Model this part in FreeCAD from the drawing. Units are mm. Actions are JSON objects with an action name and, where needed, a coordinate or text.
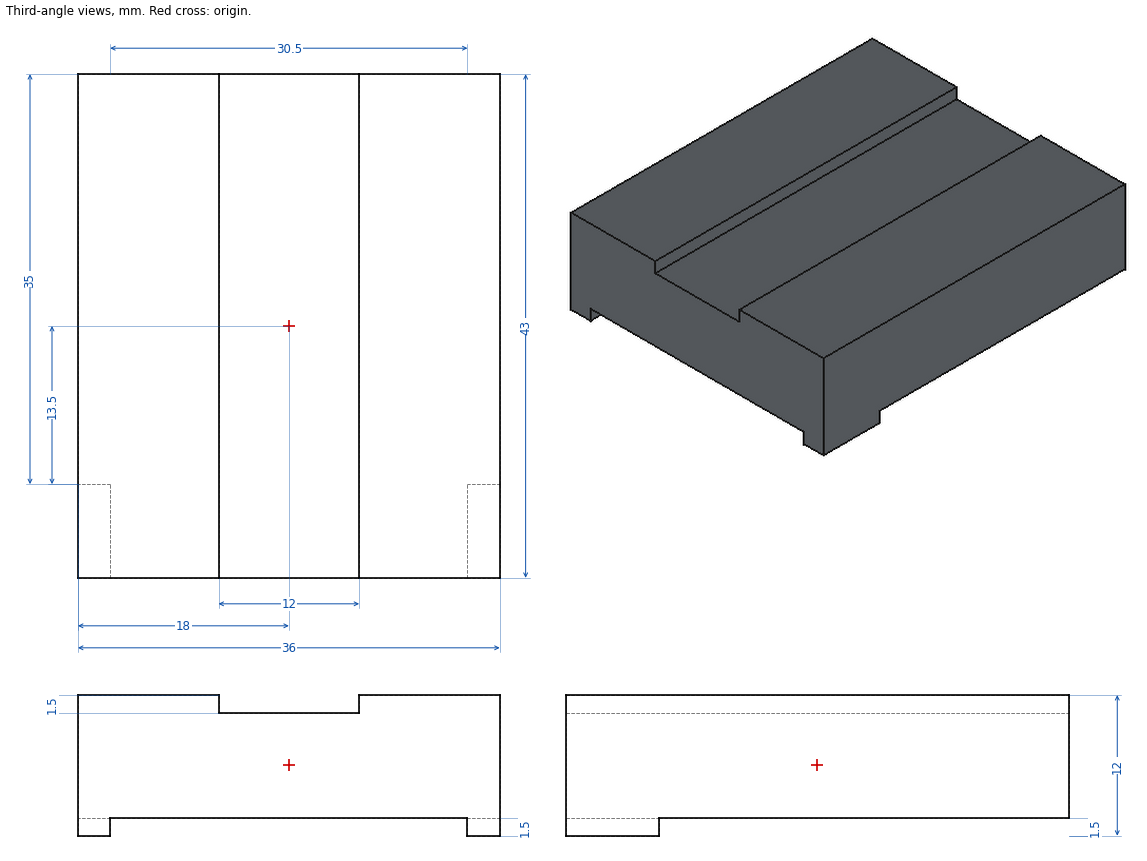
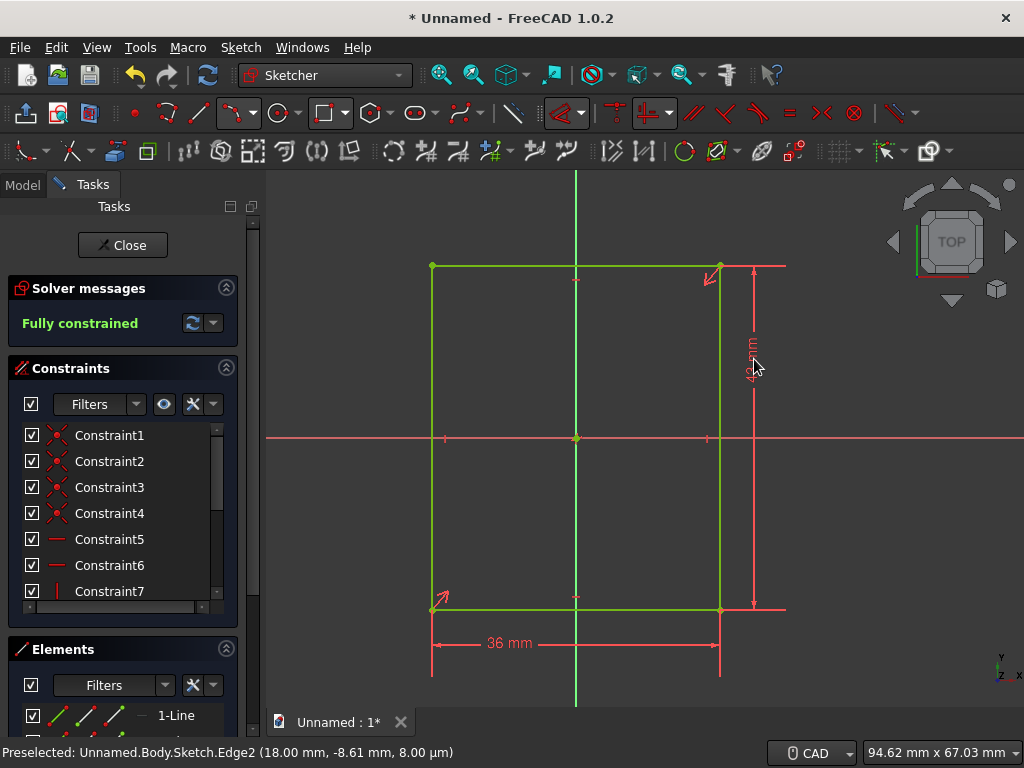
{"action": "left_click", "coordinate": [123, 245]}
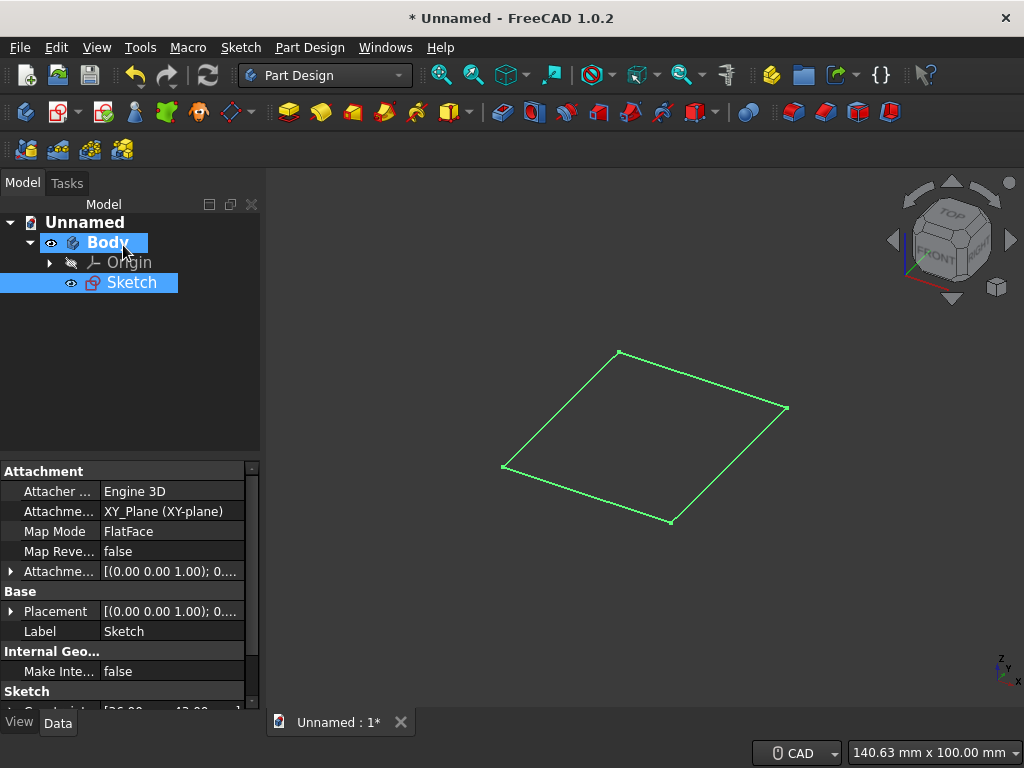
{"action": "left_click", "coordinate": [290, 112]}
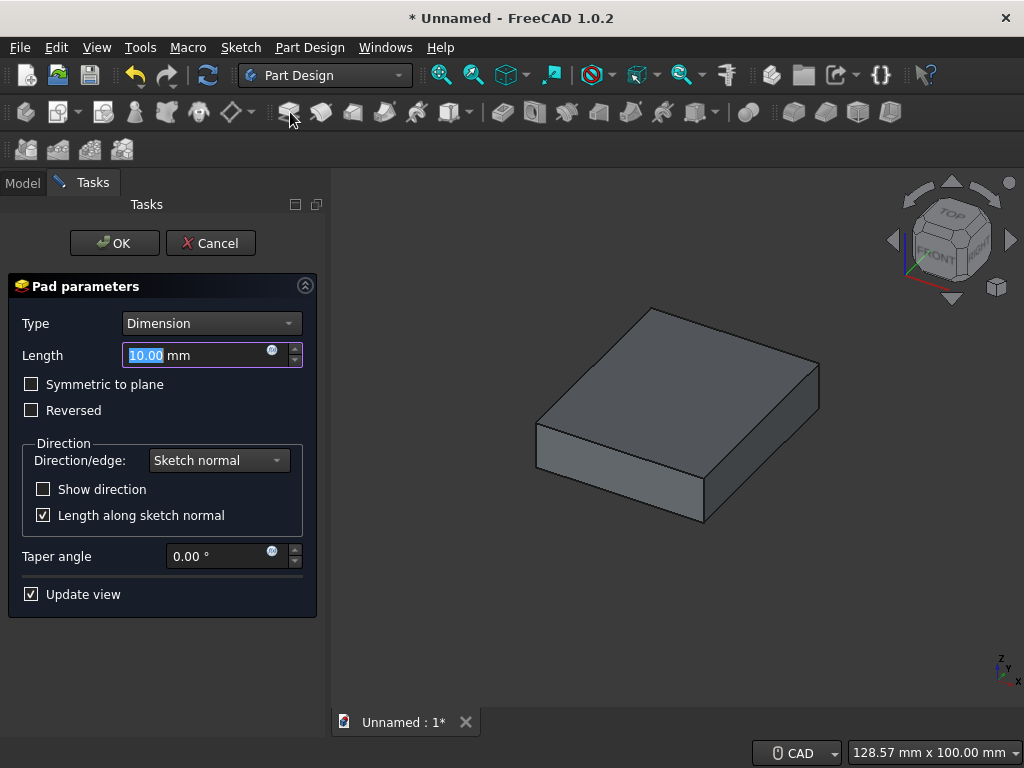
{"action": "type", "text": "12"}
{"action": "key", "text": "Tab"}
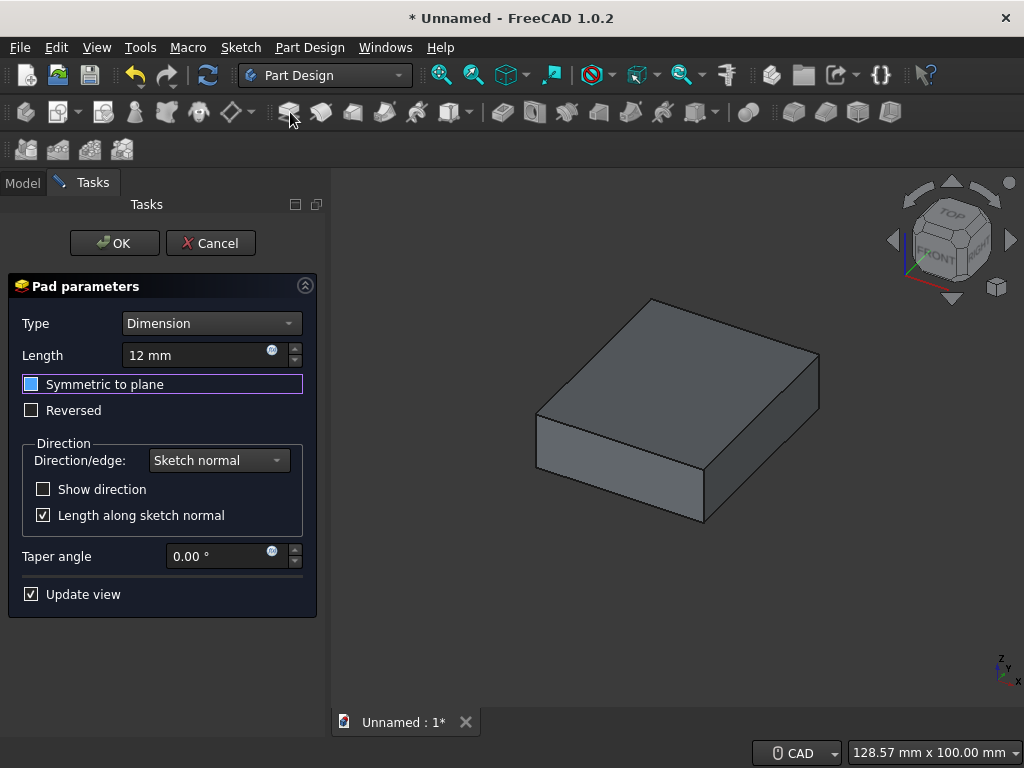
{"action": "left_click", "coordinate": [30, 384]}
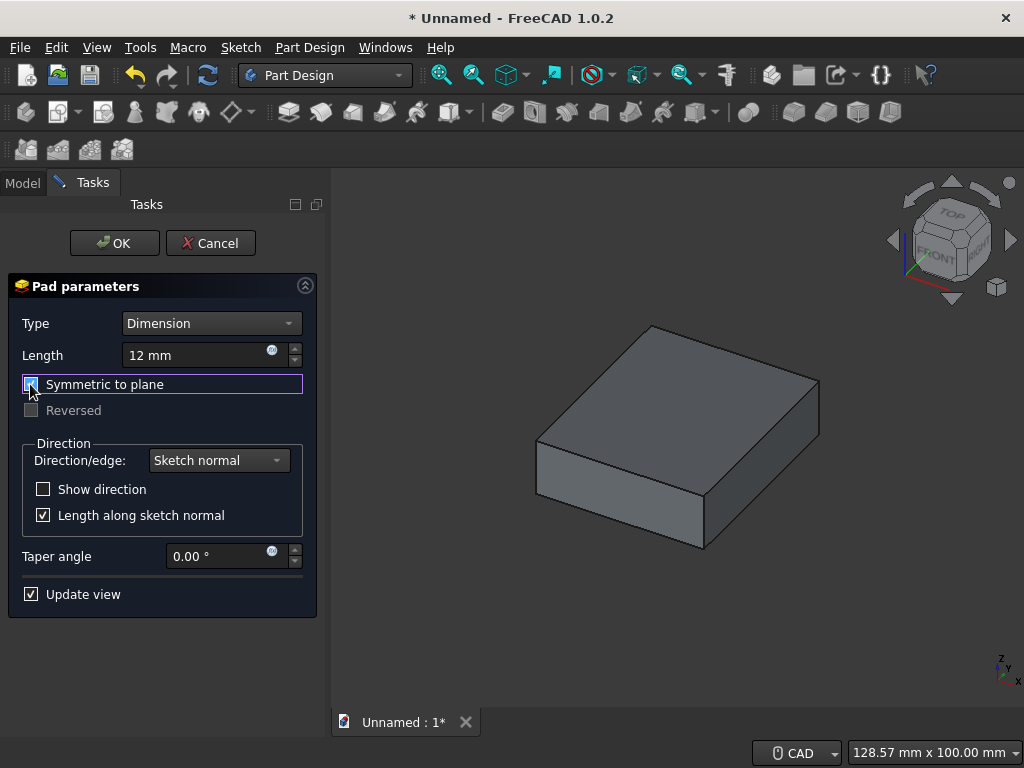
{"action": "left_click", "coordinate": [115, 243]}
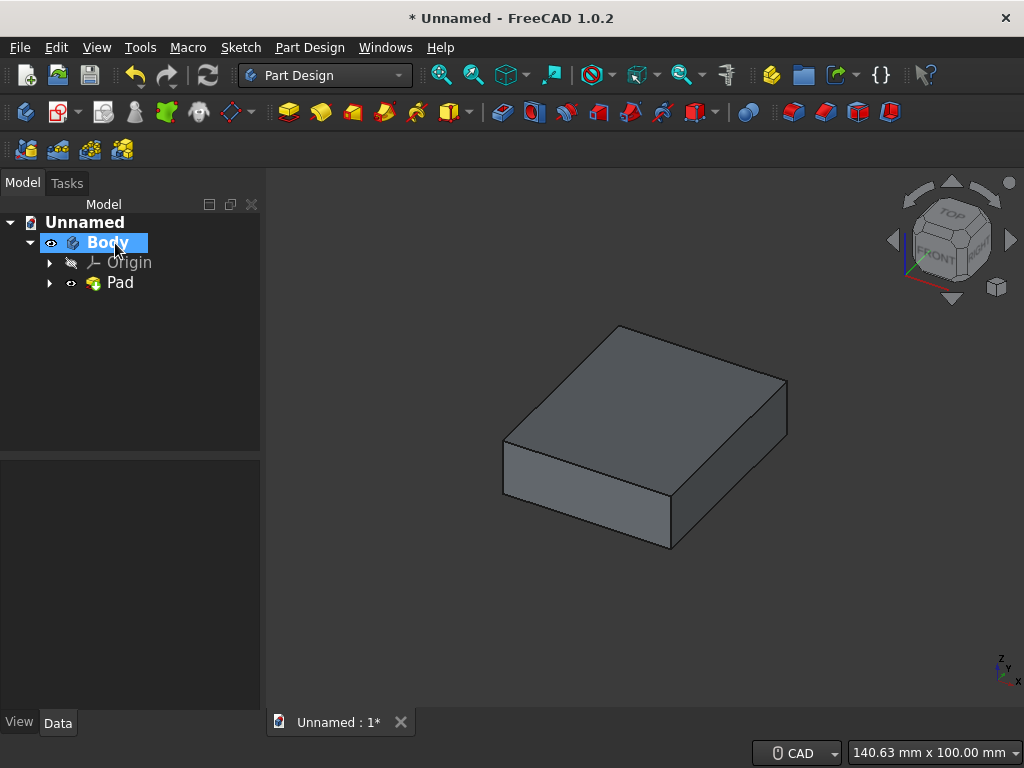
{"action": "key", "text": "v f"}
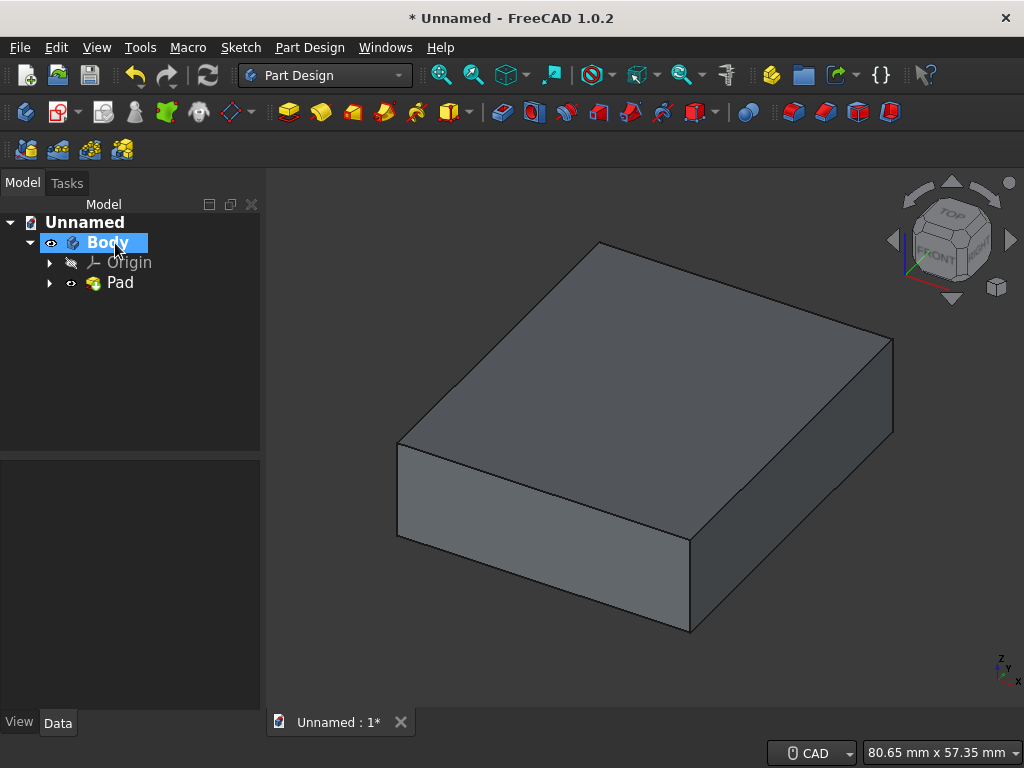
{"action": "left_click", "coordinate": [645, 390]}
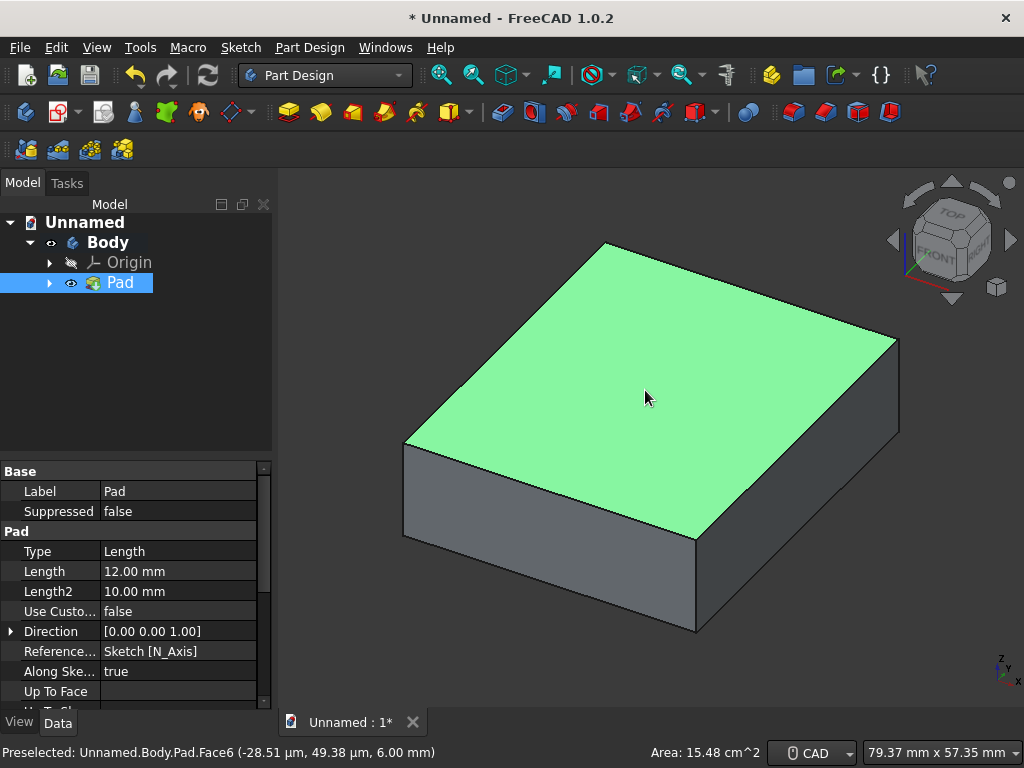
{"action": "left_click", "coordinate": [58, 112]}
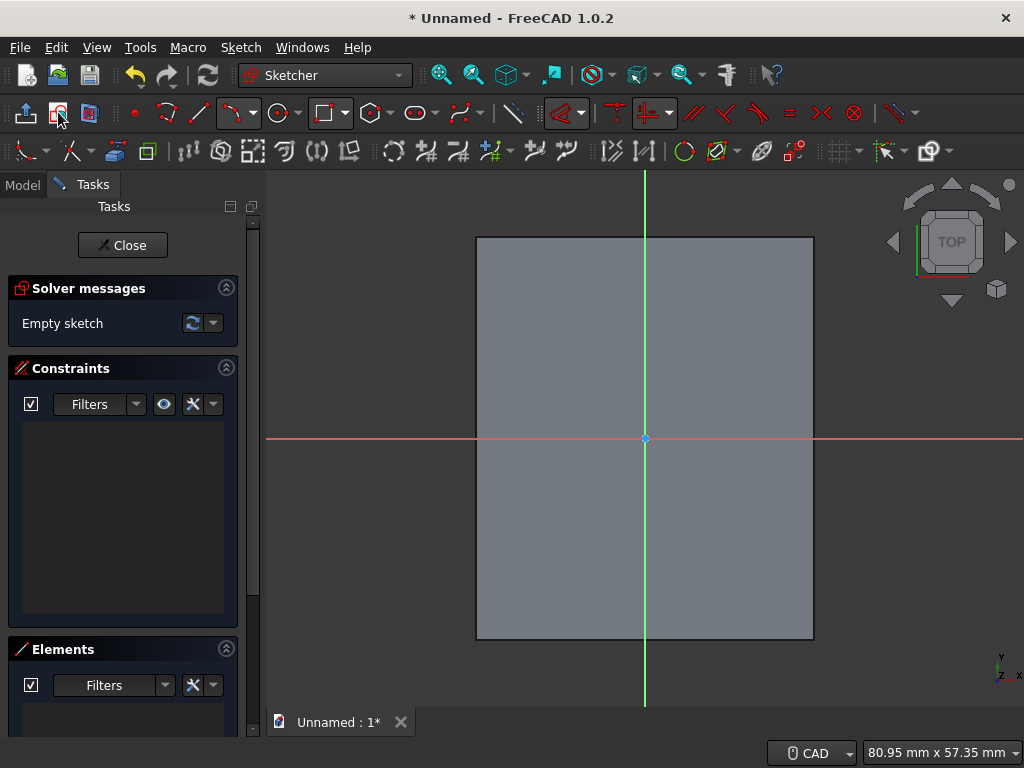
{"action": "key", "text": "g v"}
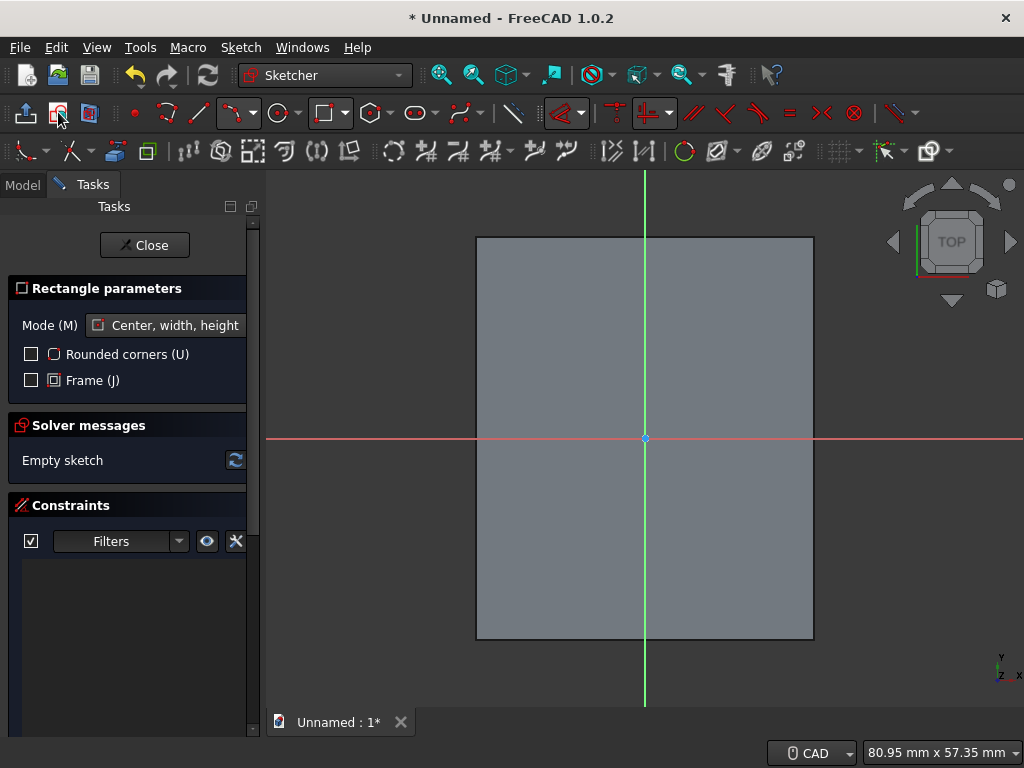
{"action": "left_click", "coordinate": [645, 438]}
{"action": "left_click", "coordinate": [701, 237]}
{"action": "key", "text": "Escape"}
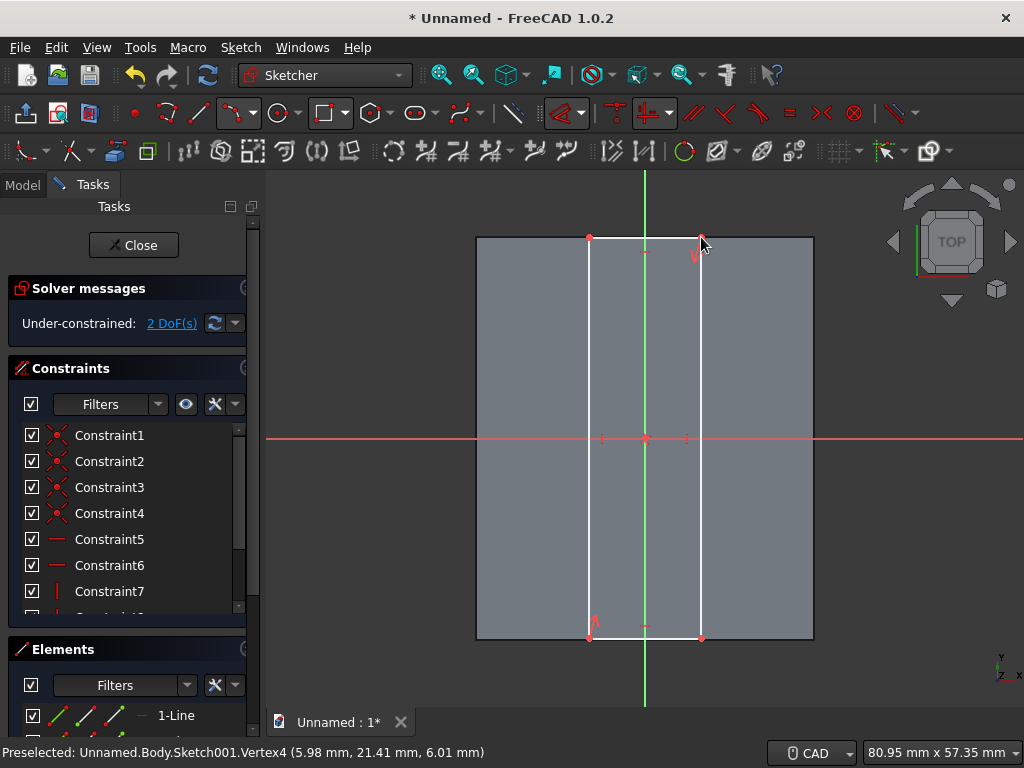
{"action": "key", "text": "d"}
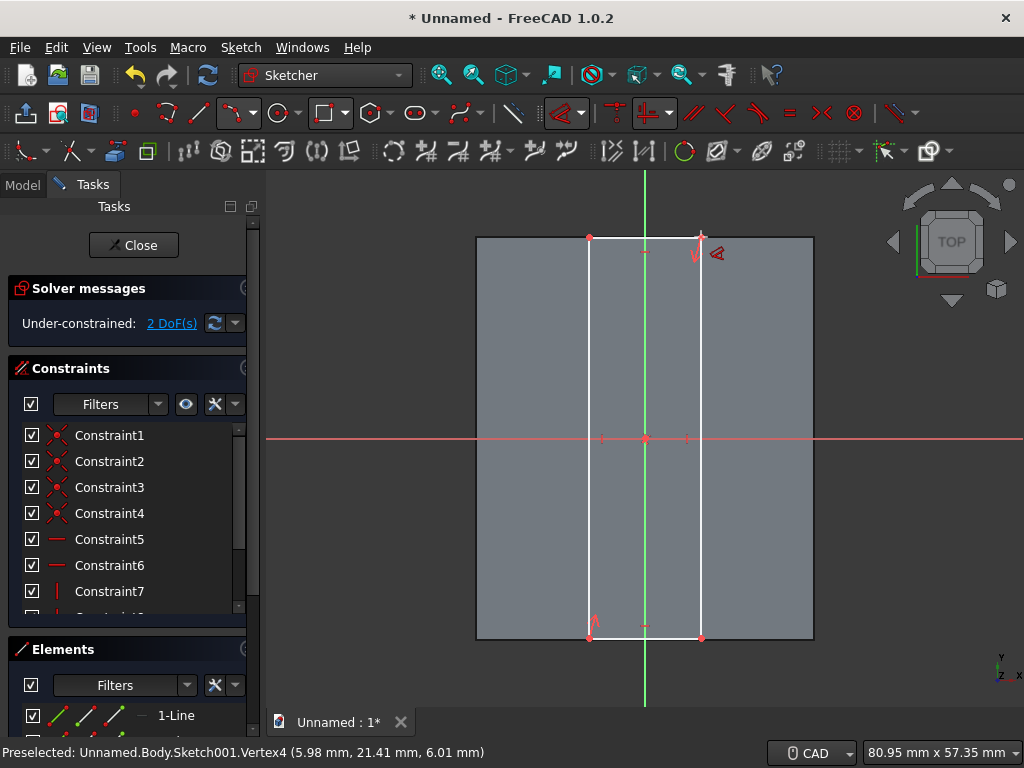
{"action": "left_click", "coordinate": [623, 639]}
{"action": "left_click", "coordinate": [619, 673]}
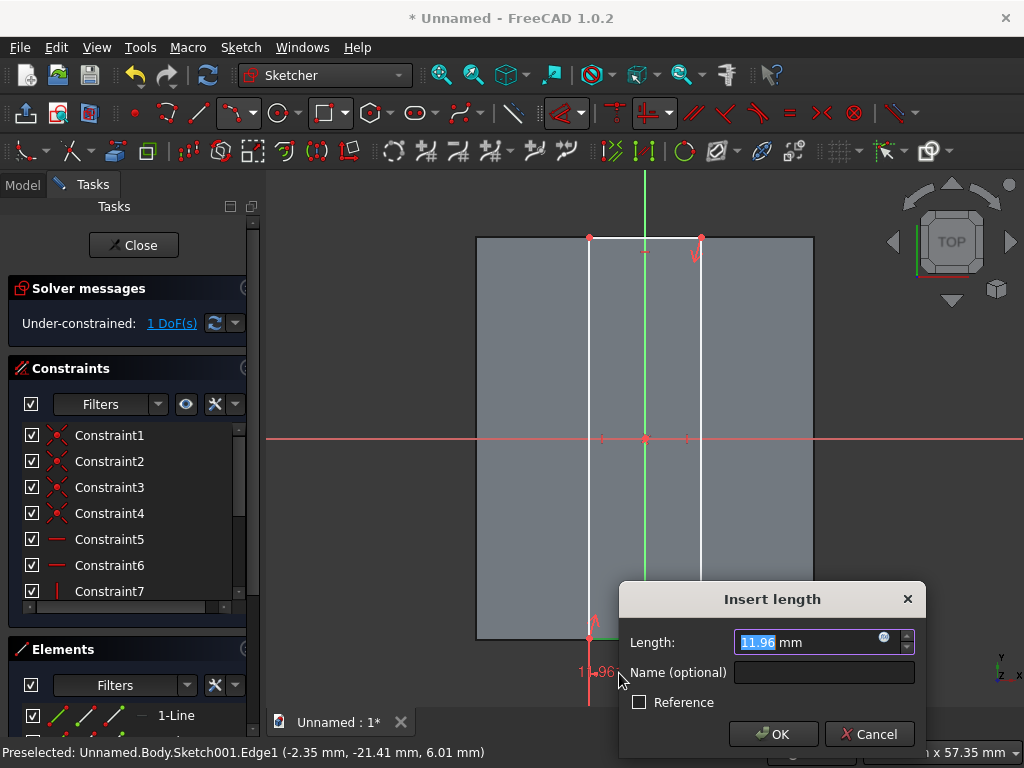
{"action": "type", "text": "12"}
{"action": "key", "text": "Return"}